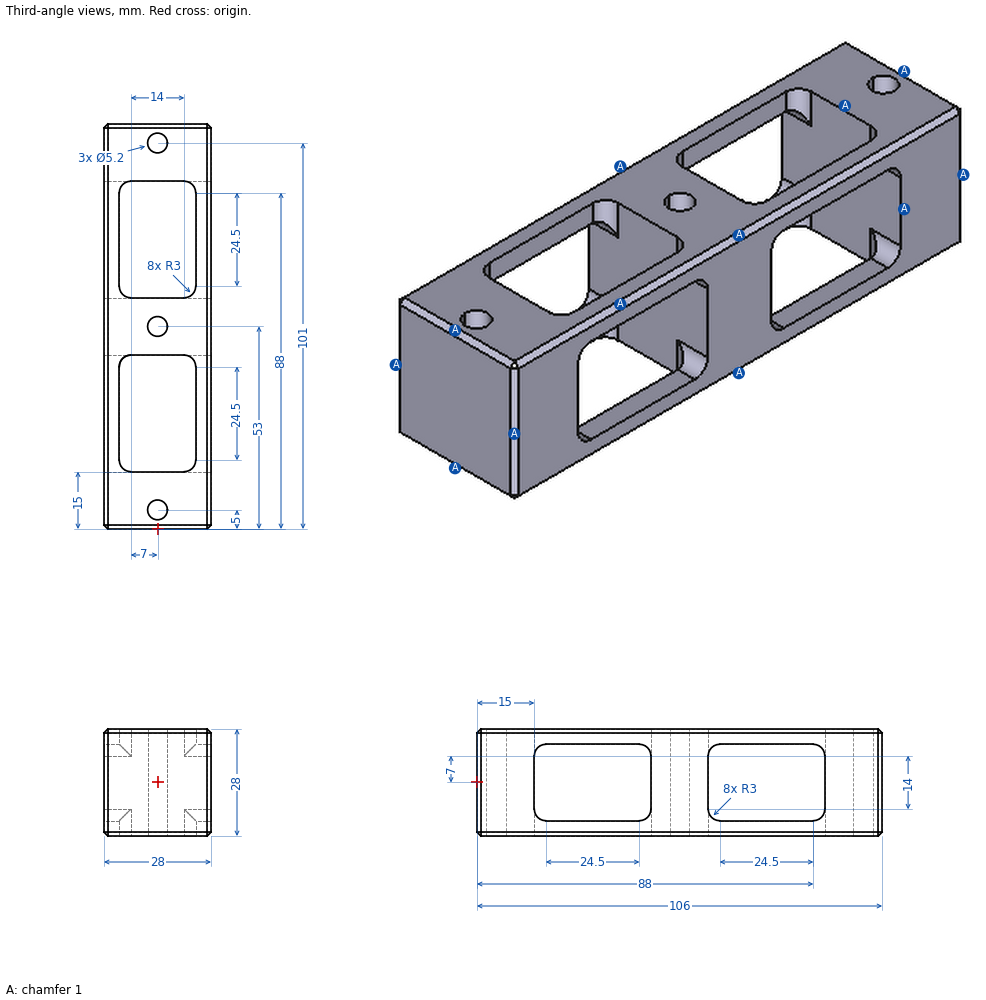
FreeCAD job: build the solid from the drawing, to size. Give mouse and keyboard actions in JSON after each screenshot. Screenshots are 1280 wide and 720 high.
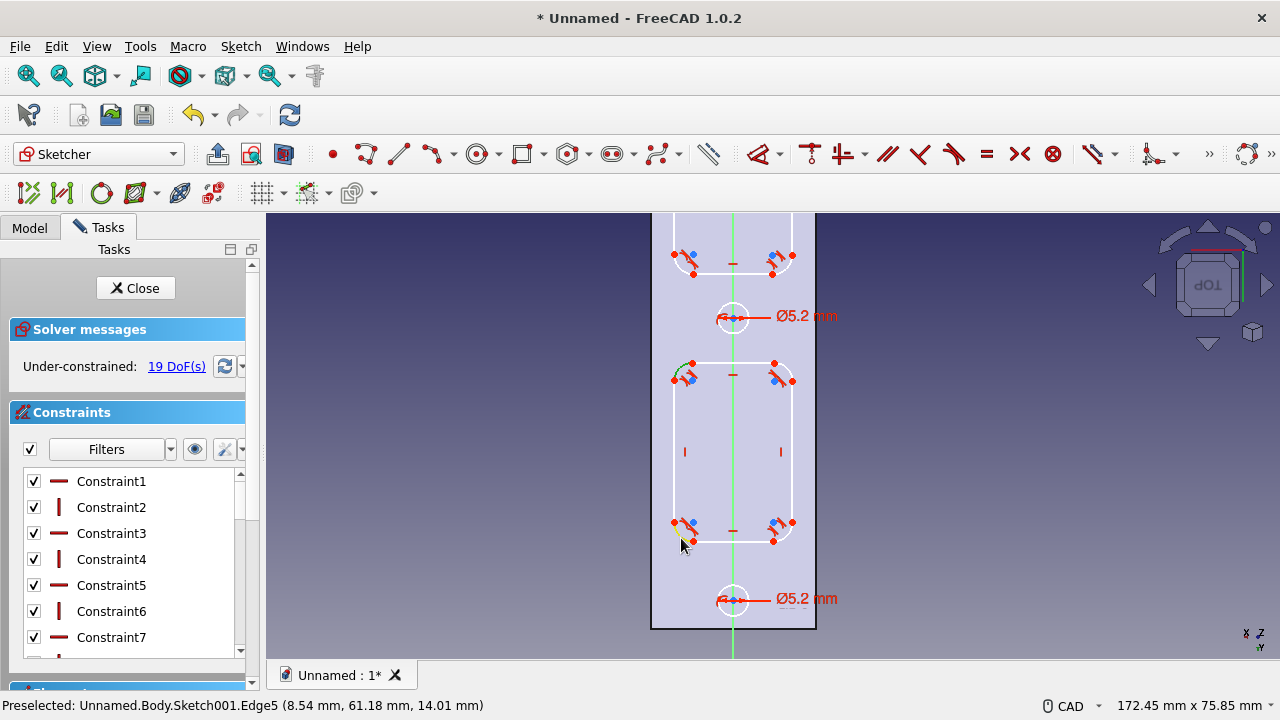
{"action": "left_click", "coordinate": [680, 536]}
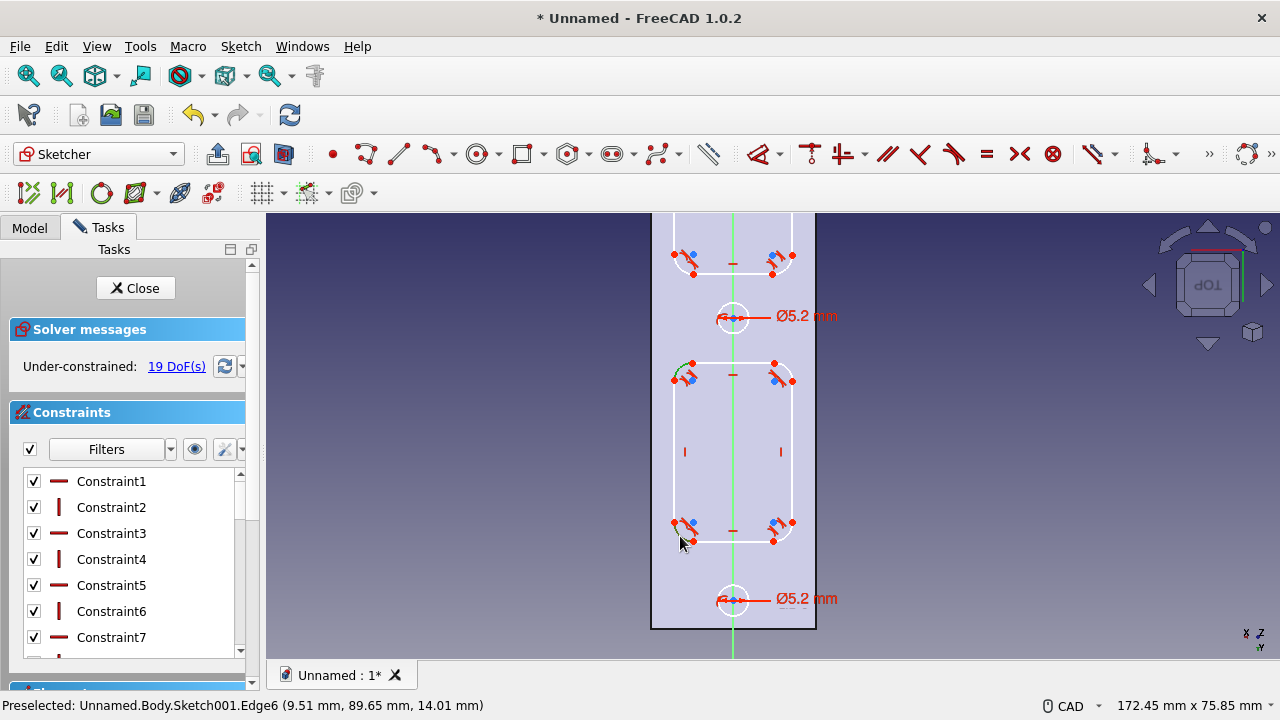
{"action": "scroll", "coordinate": [782, 539], "scroll_direction": "up", "scroll_amount": 3}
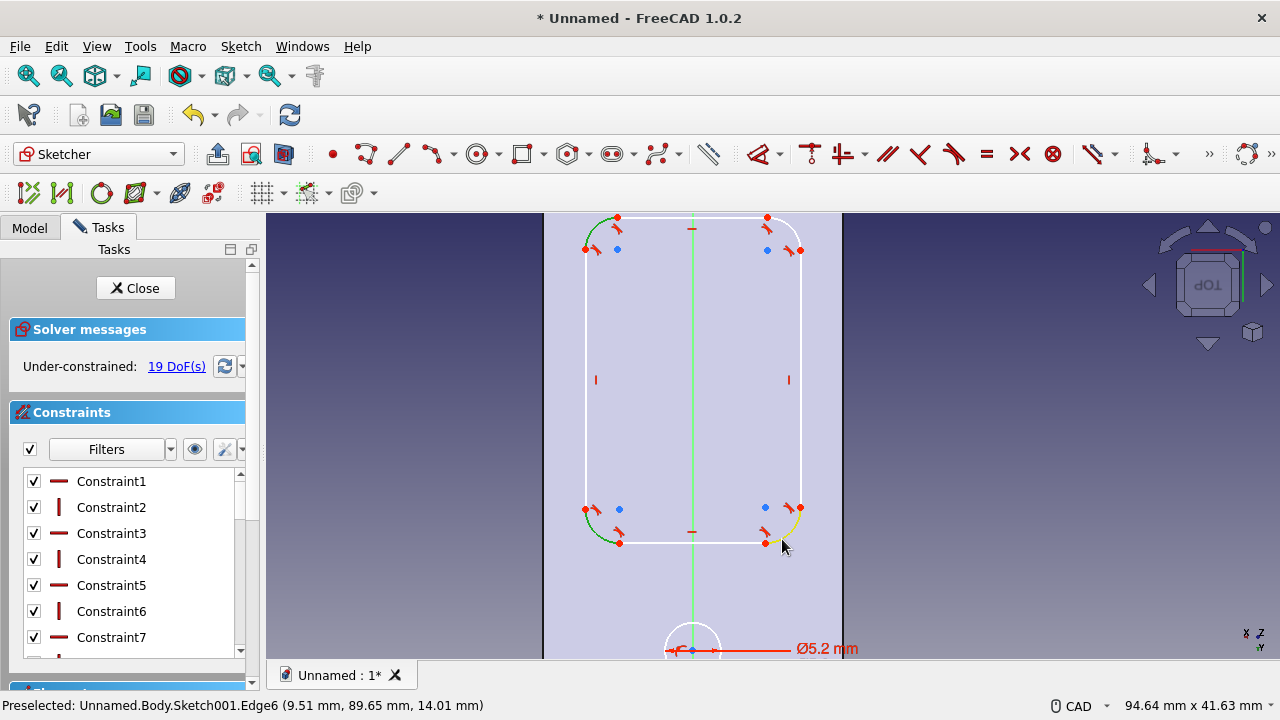
{"action": "left_click", "coordinate": [781, 539]}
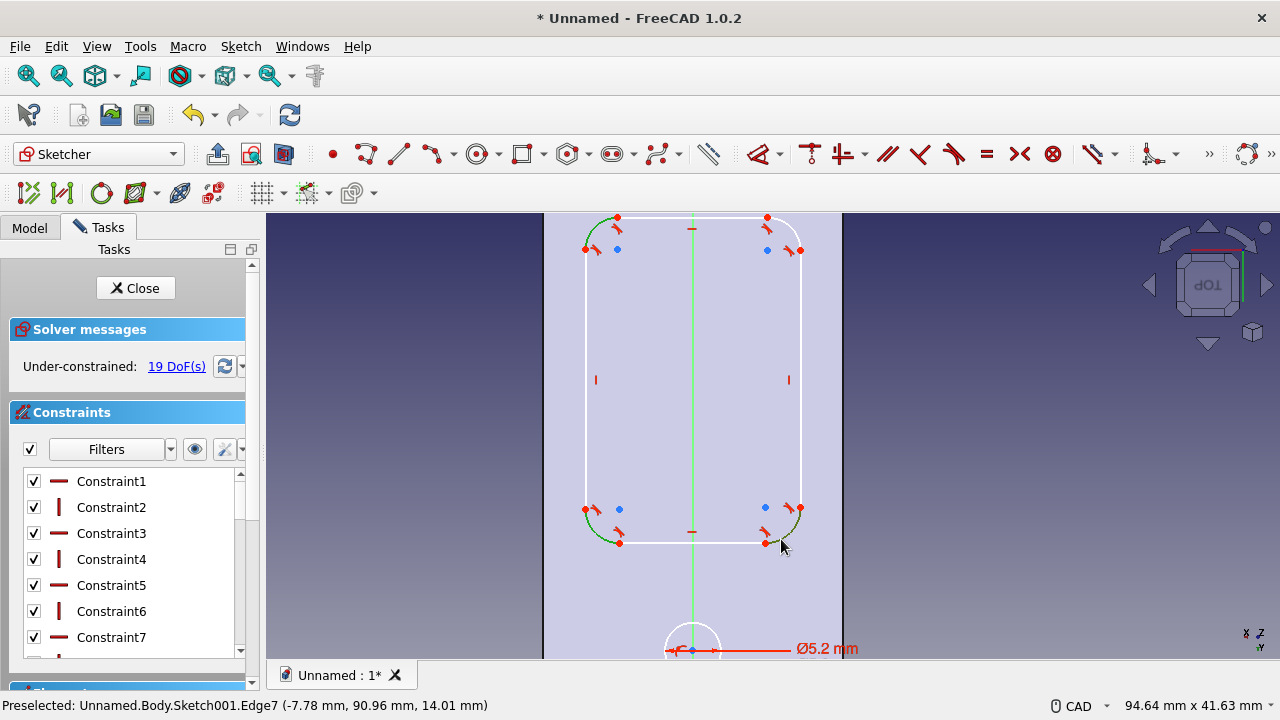
{"action": "scroll", "coordinate": [708, 539], "scroll_direction": "down", "scroll_amount": 7}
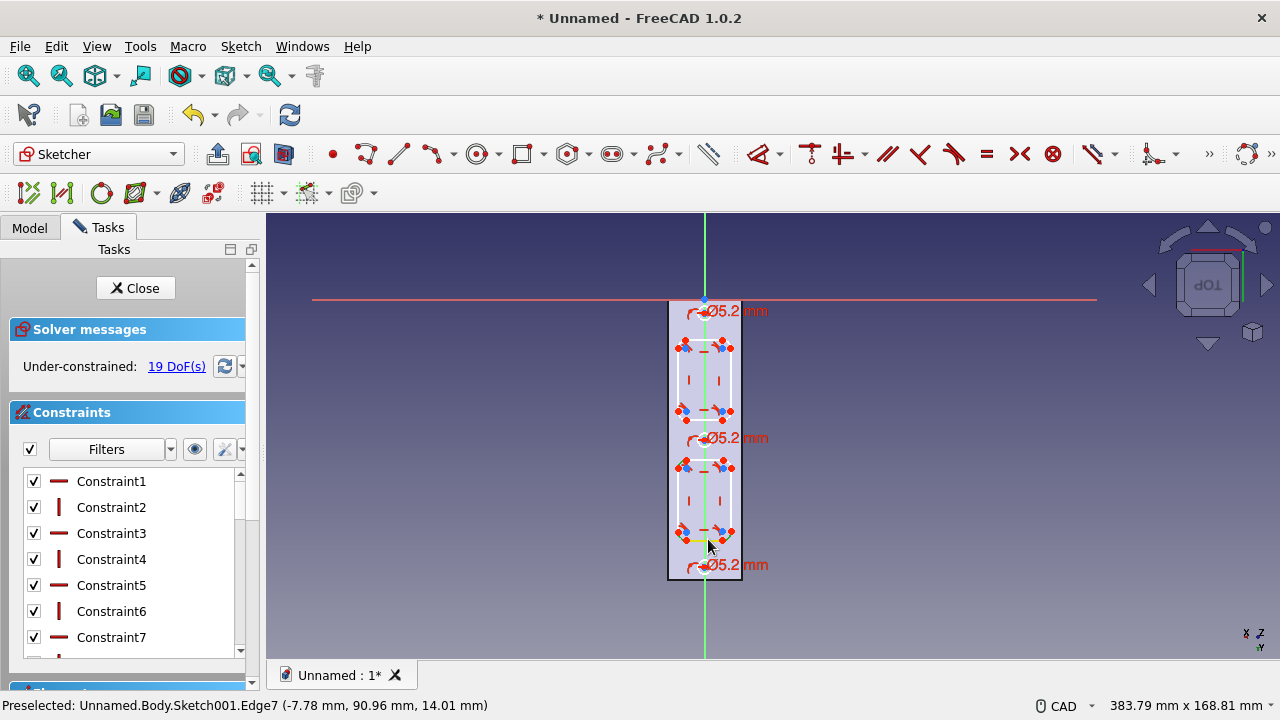
{"action": "scroll", "coordinate": [730, 465], "scroll_direction": "up", "scroll_amount": 7}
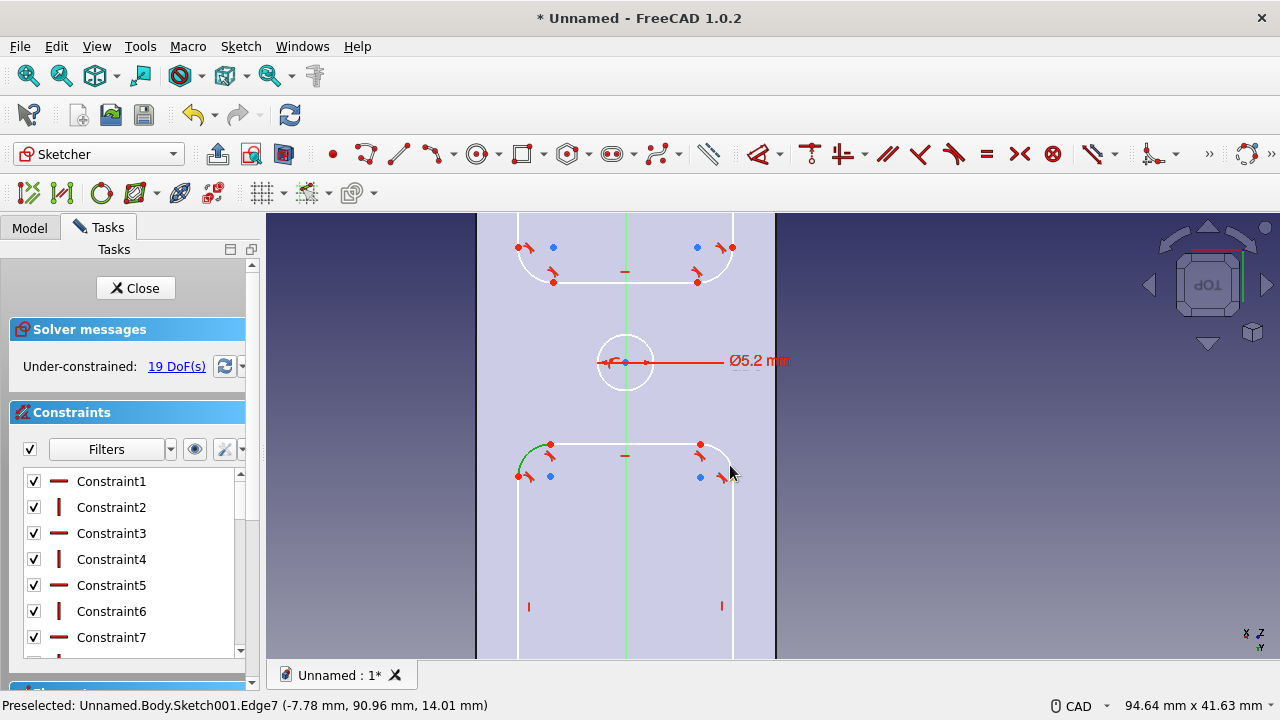
{"action": "left_click", "coordinate": [730, 462]}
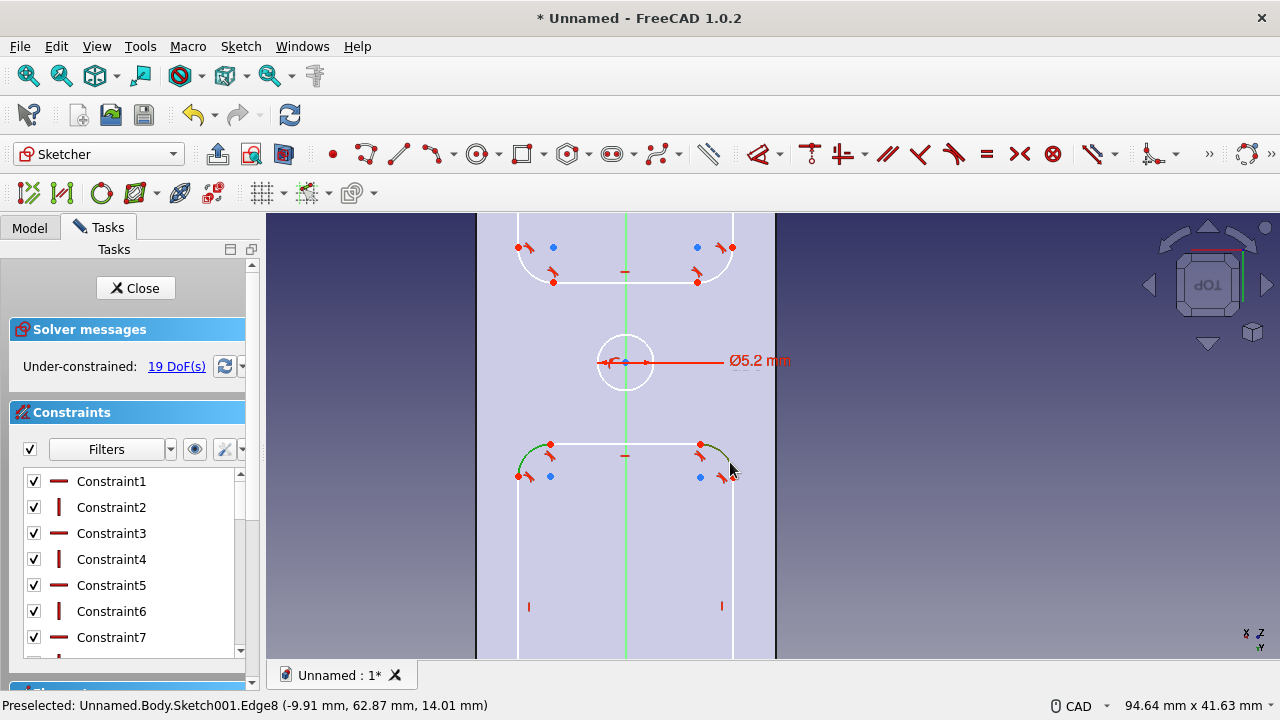
{"action": "scroll", "coordinate": [730, 465], "scroll_direction": "down", "scroll_amount": 7}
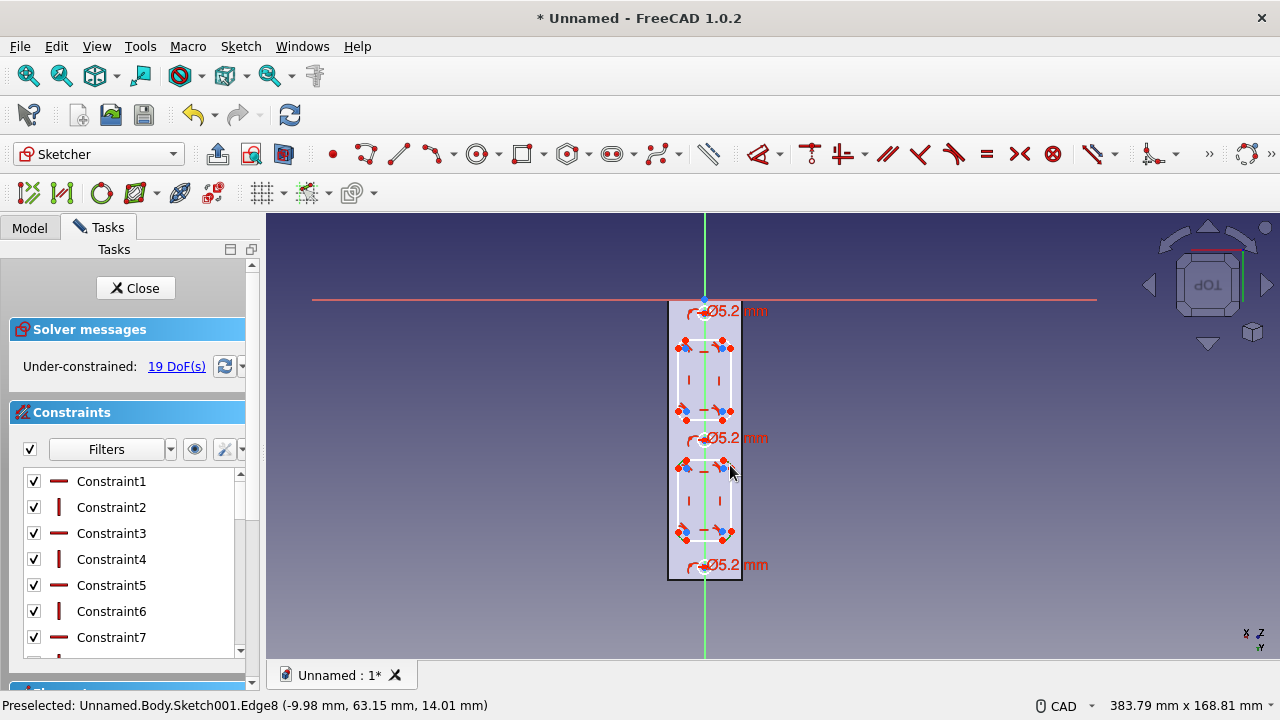
{"action": "scroll", "coordinate": [682, 341], "scroll_direction": "up", "scroll_amount": 7}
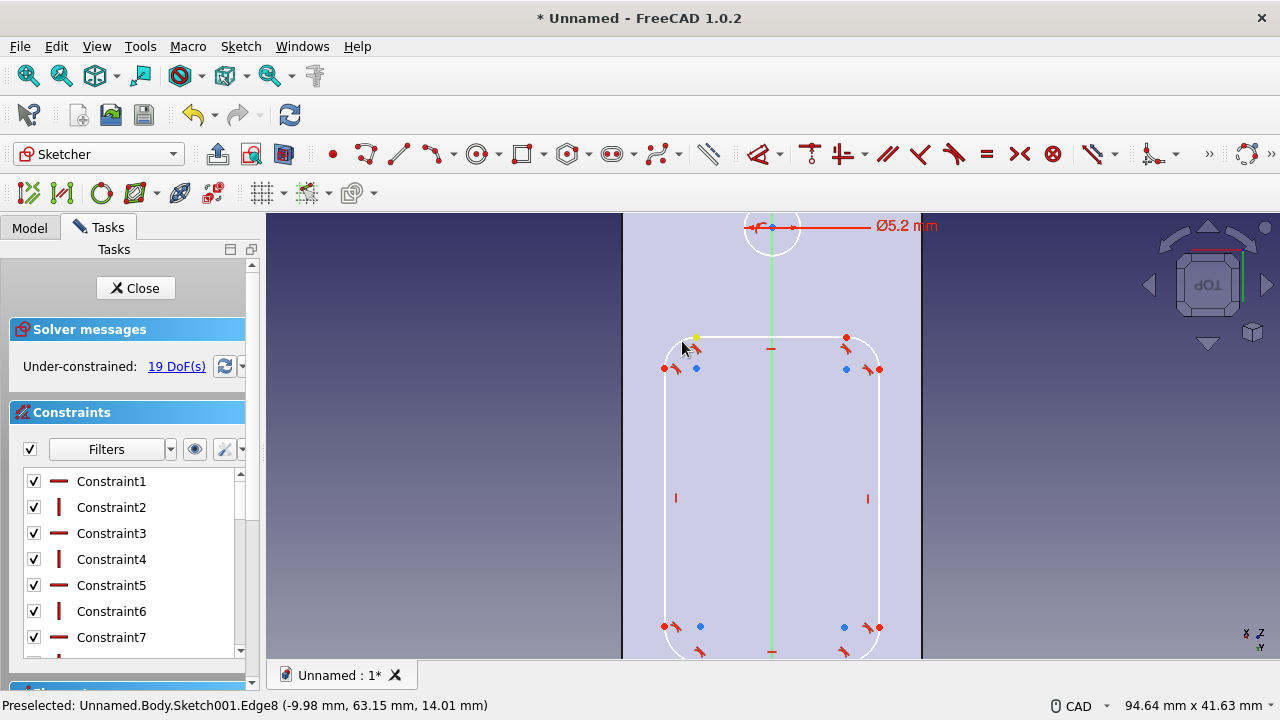
{"action": "left_click", "coordinate": [682, 341]}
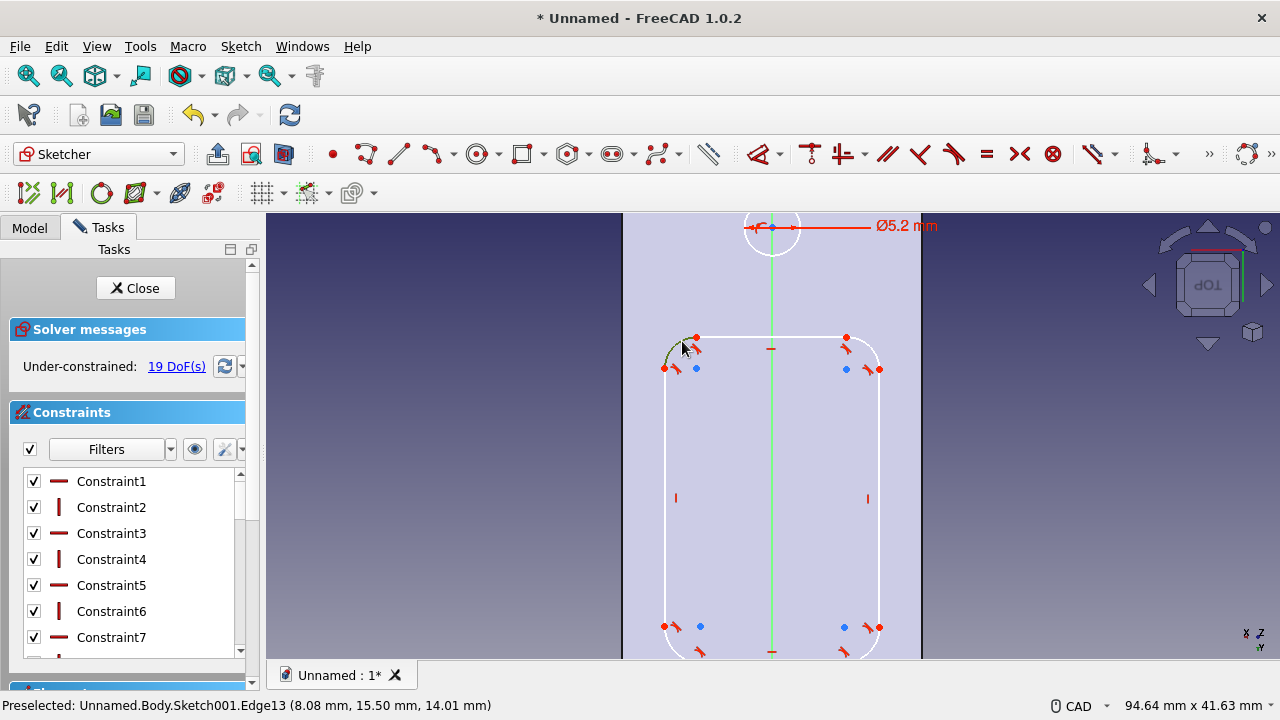
{"action": "scroll", "coordinate": [682, 340], "scroll_direction": "down", "scroll_amount": 7}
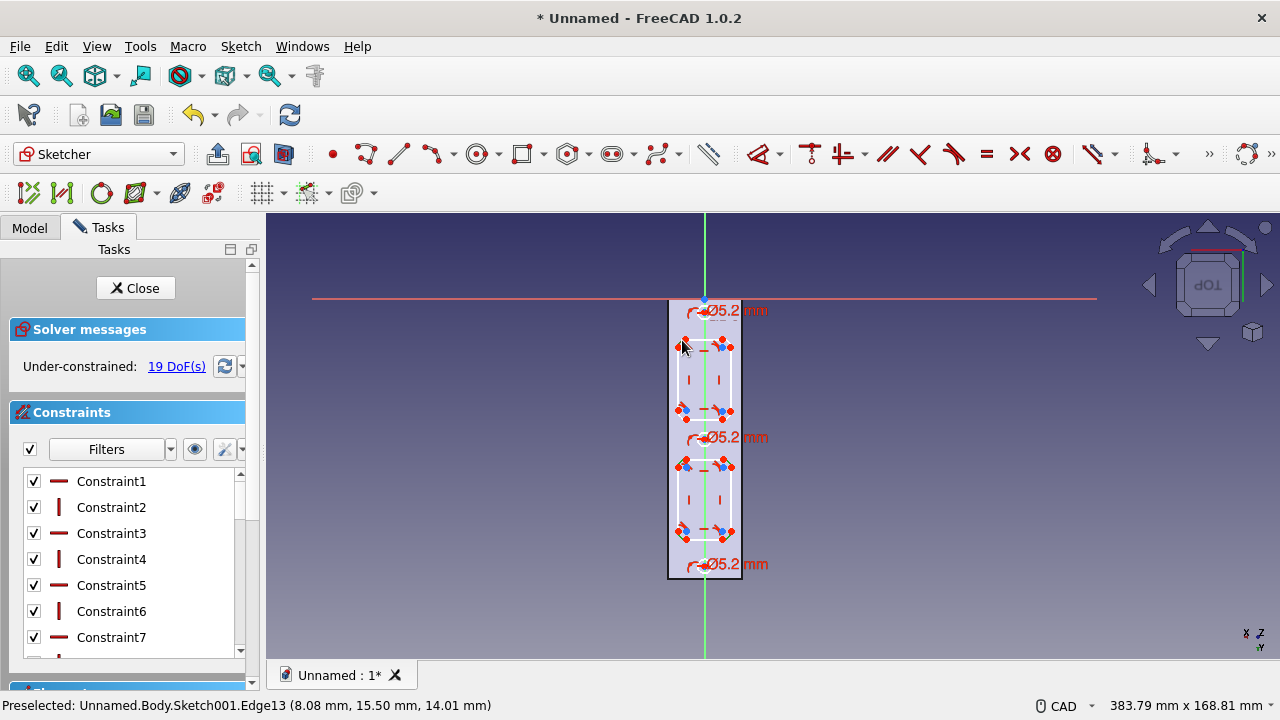
{"action": "scroll", "coordinate": [679, 415], "scroll_direction": "up", "scroll_amount": 7}